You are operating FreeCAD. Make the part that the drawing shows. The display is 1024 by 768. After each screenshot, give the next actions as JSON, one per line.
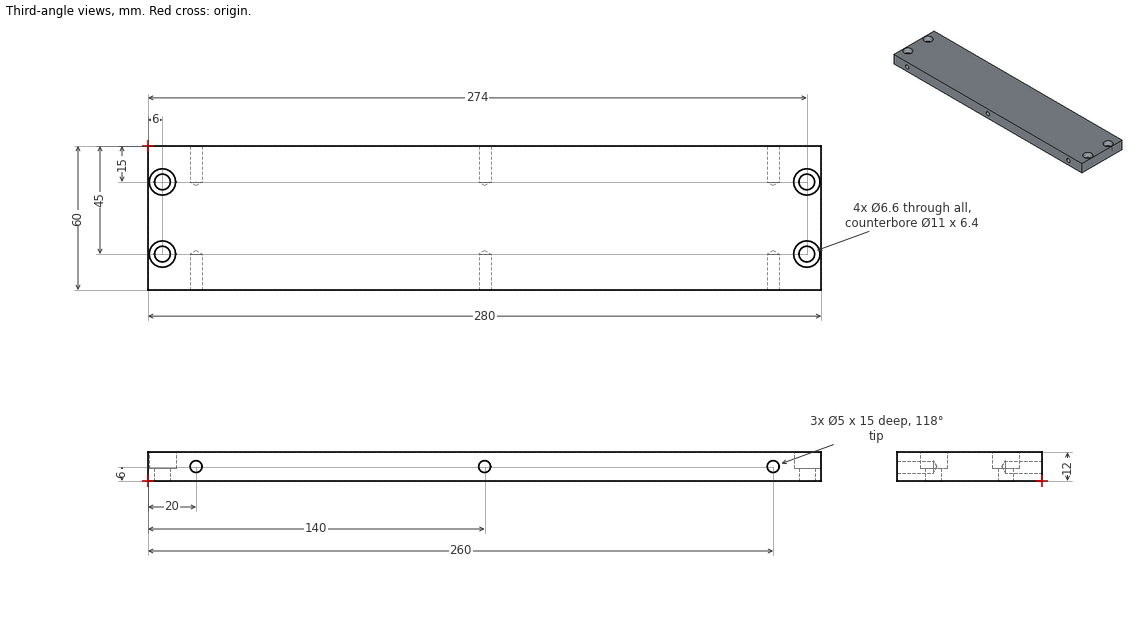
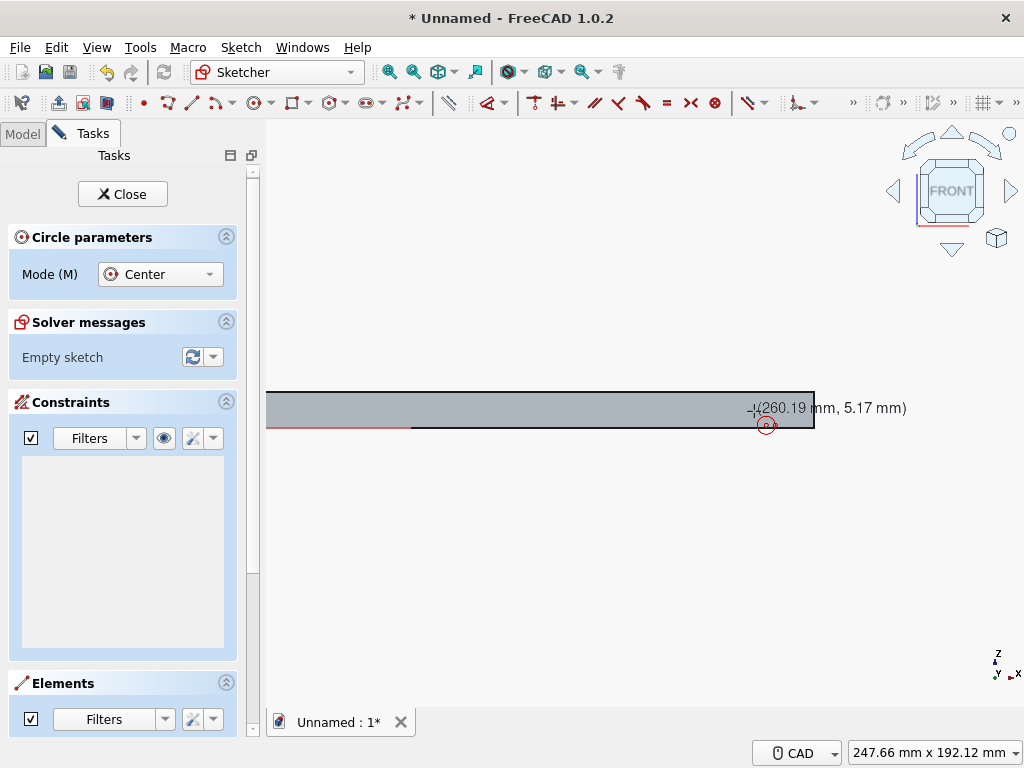
{"action": "left_click", "coordinate": [753, 410]}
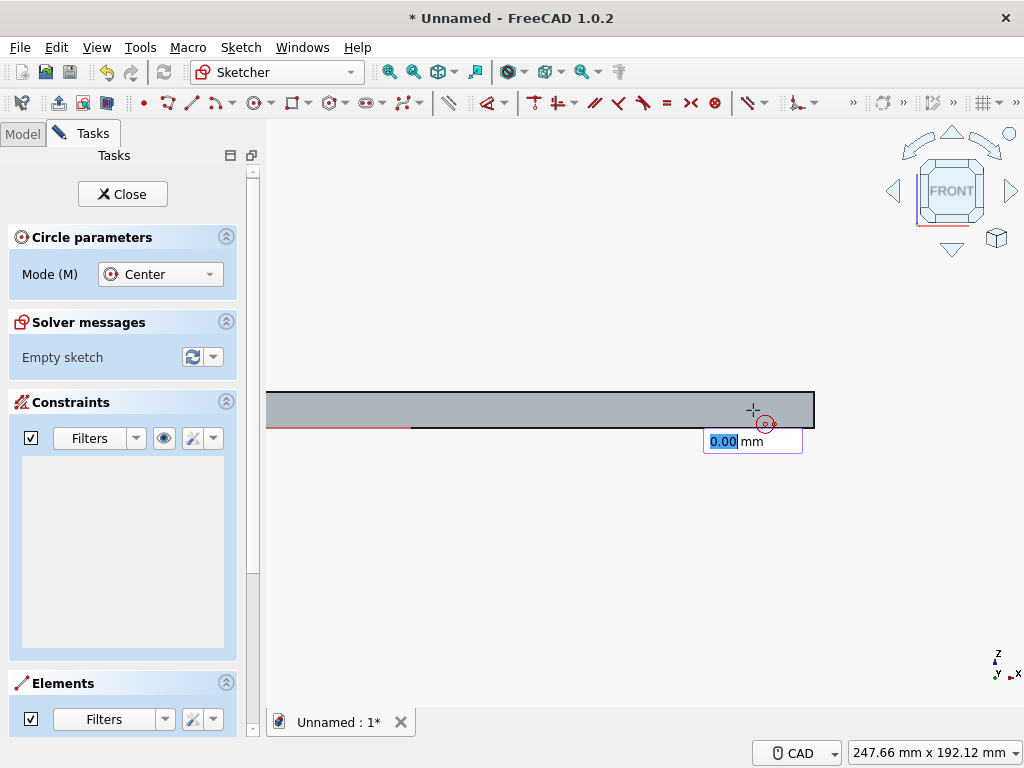
{"action": "scroll", "coordinate": [758, 405], "scroll_direction": "up", "scroll_amount": 4}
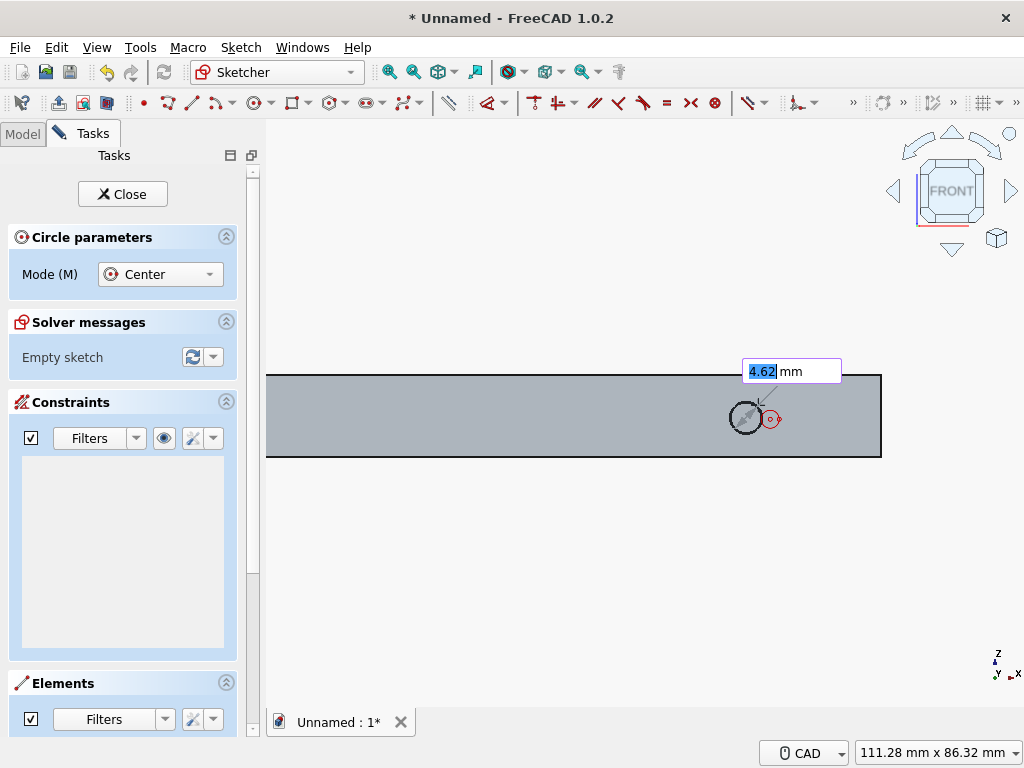
{"action": "left_click", "coordinate": [757, 404]}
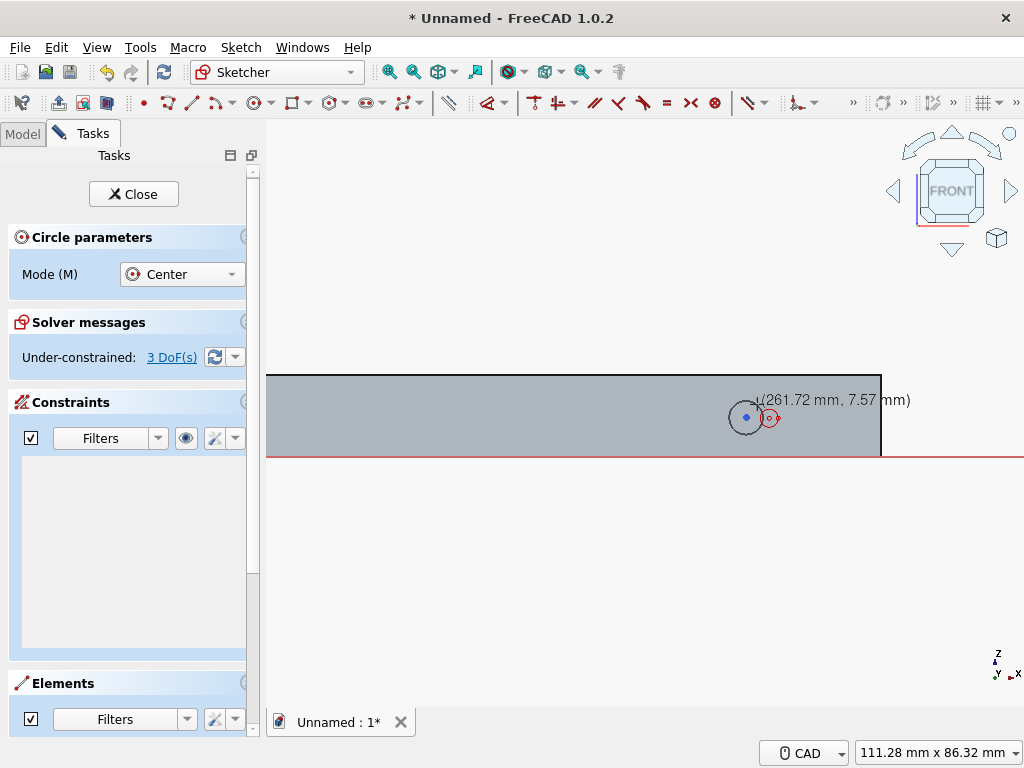
{"action": "scroll", "coordinate": [756, 409], "scroll_direction": "down", "scroll_amount": 8}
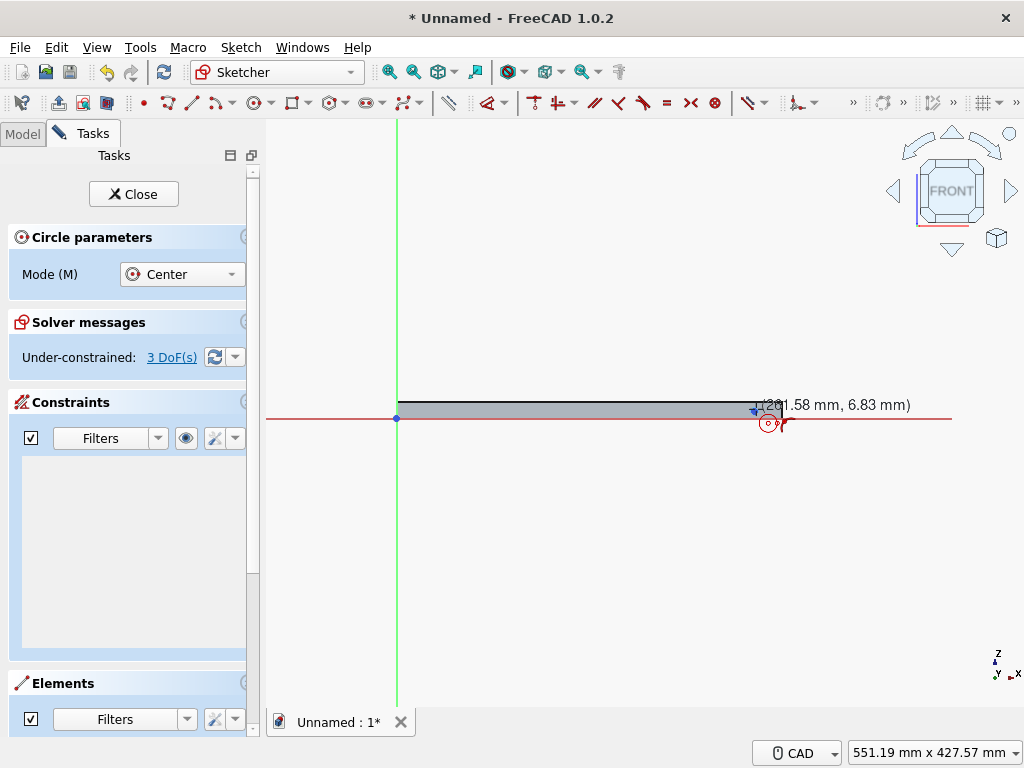
{"action": "scroll", "coordinate": [589, 411], "scroll_direction": "up", "scroll_amount": 10}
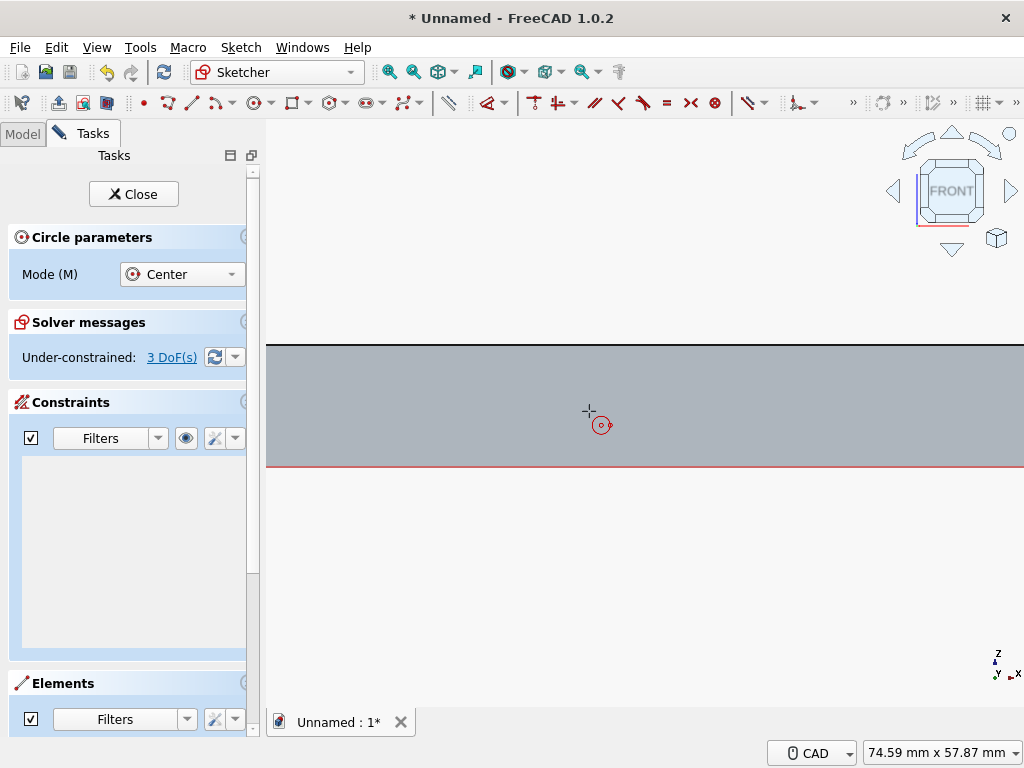
{"action": "scroll", "coordinate": [589, 411], "scroll_direction": "down", "scroll_amount": 10}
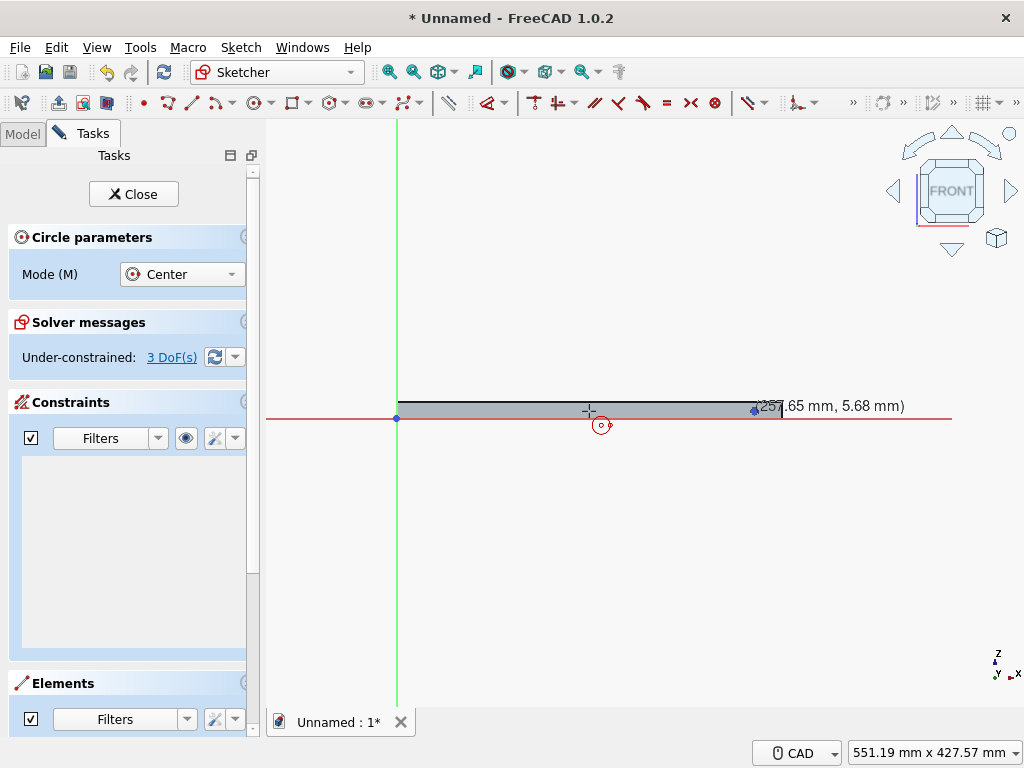
{"action": "scroll", "coordinate": [589, 411], "scroll_direction": "up", "scroll_amount": 4}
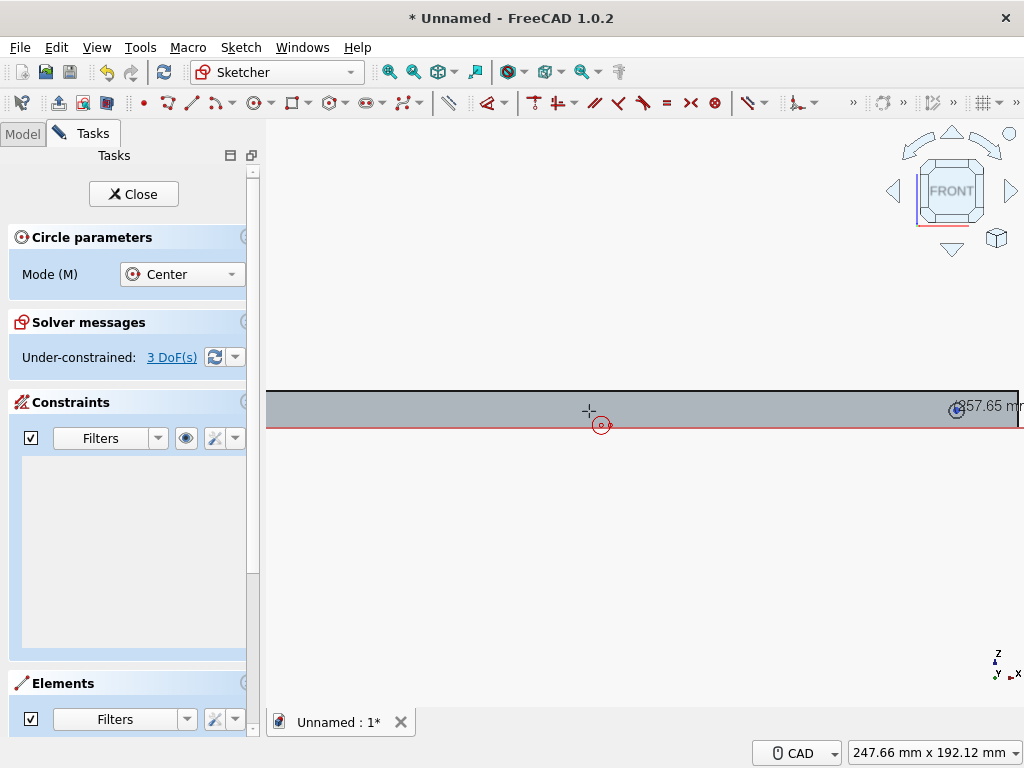
{"action": "left_click", "coordinate": [589, 410]}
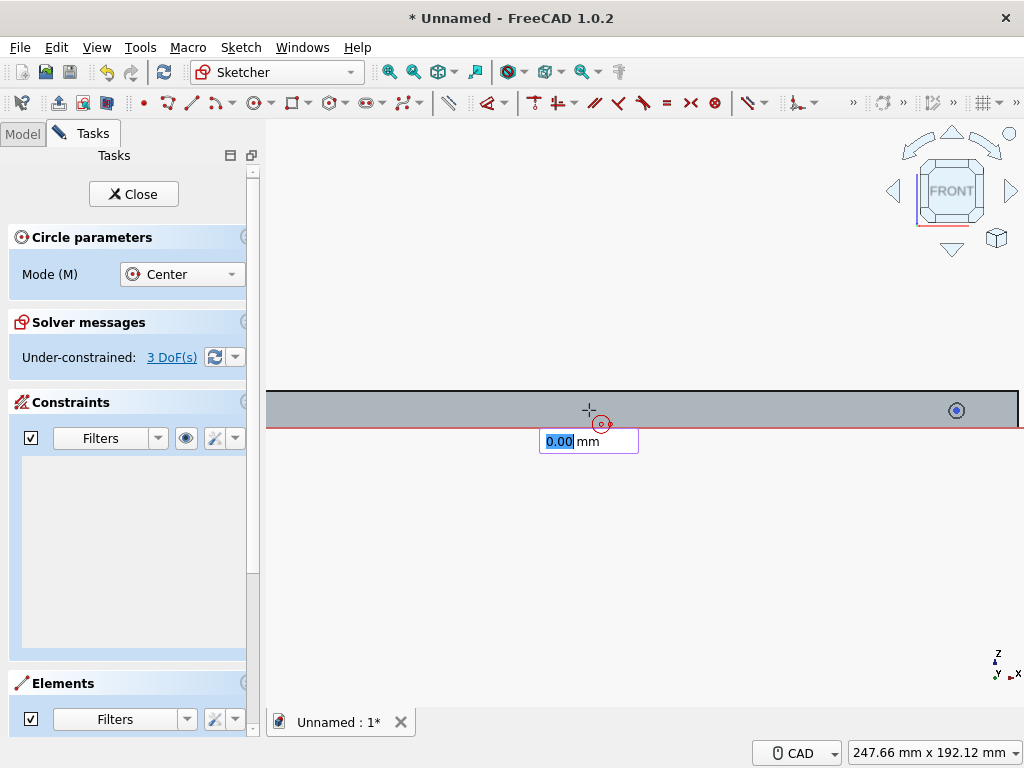
{"action": "scroll", "coordinate": [595, 404], "scroll_direction": "up", "scroll_amount": 4}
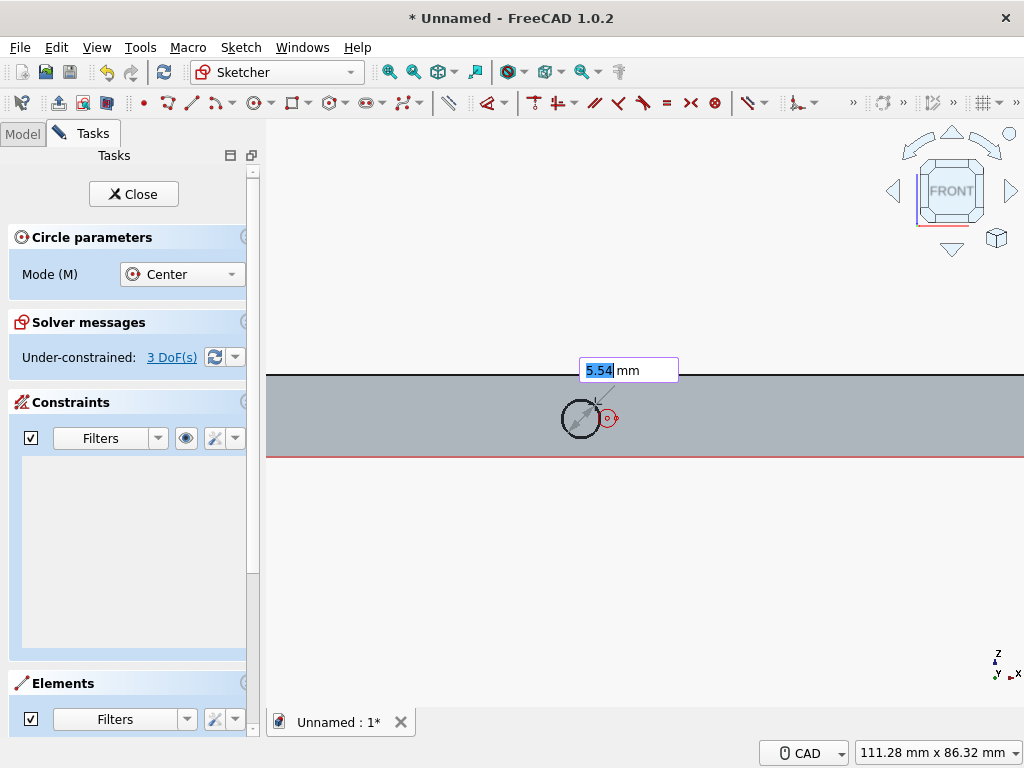
{"action": "left_click", "coordinate": [594, 404]}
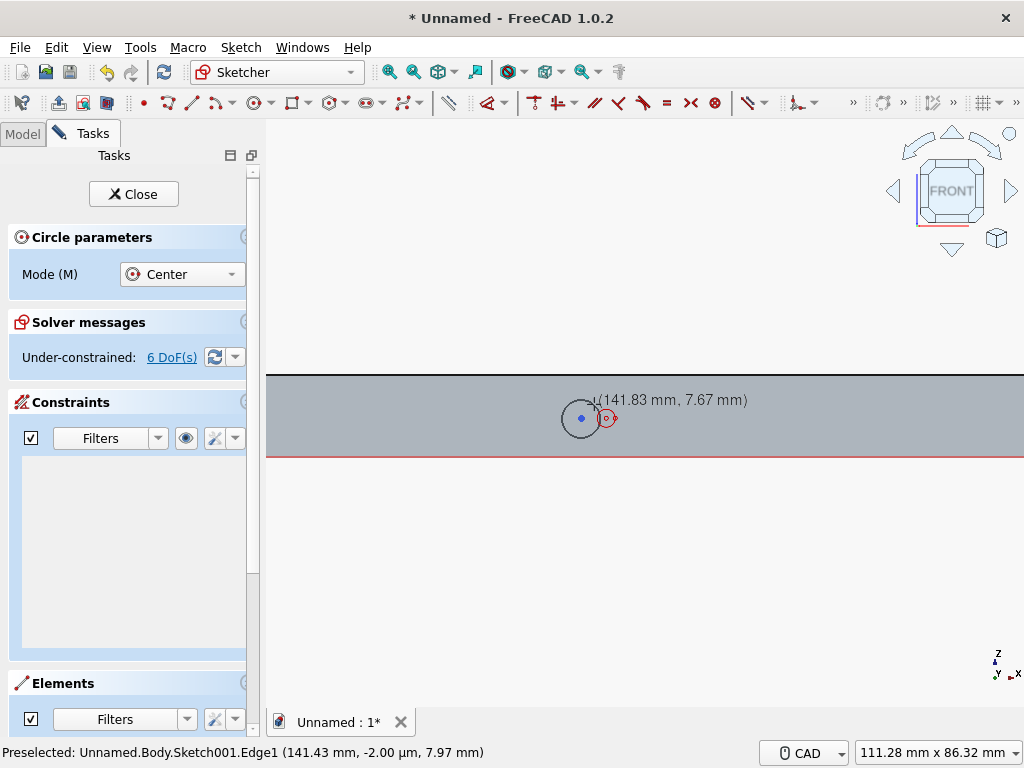
{"action": "scroll", "coordinate": [590, 409], "scroll_direction": "down", "scroll_amount": 8}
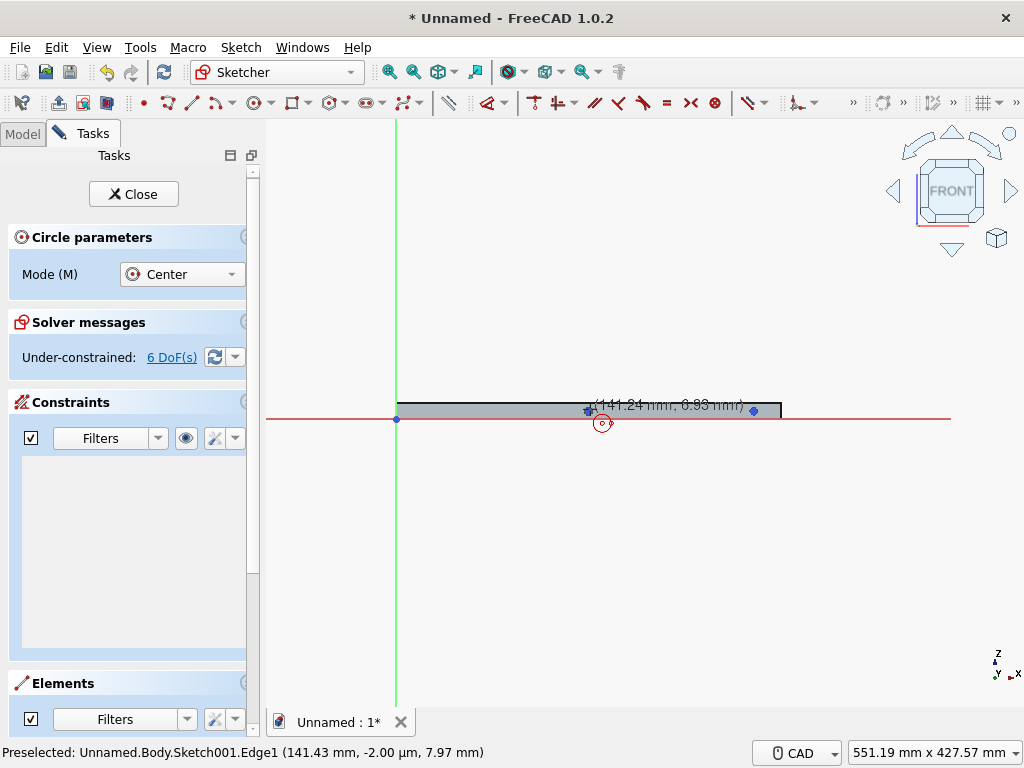
{"action": "scroll", "coordinate": [424, 411], "scroll_direction": "up", "scroll_amount": 10}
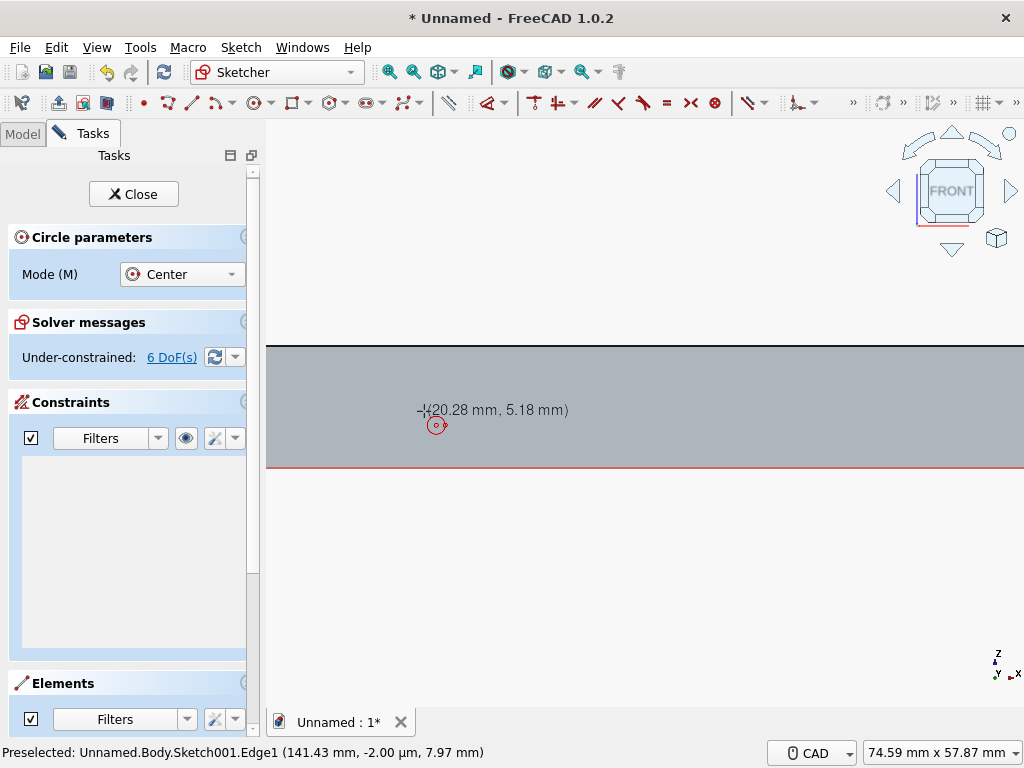
{"action": "scroll", "coordinate": [424, 411], "scroll_direction": "down", "scroll_amount": 10}